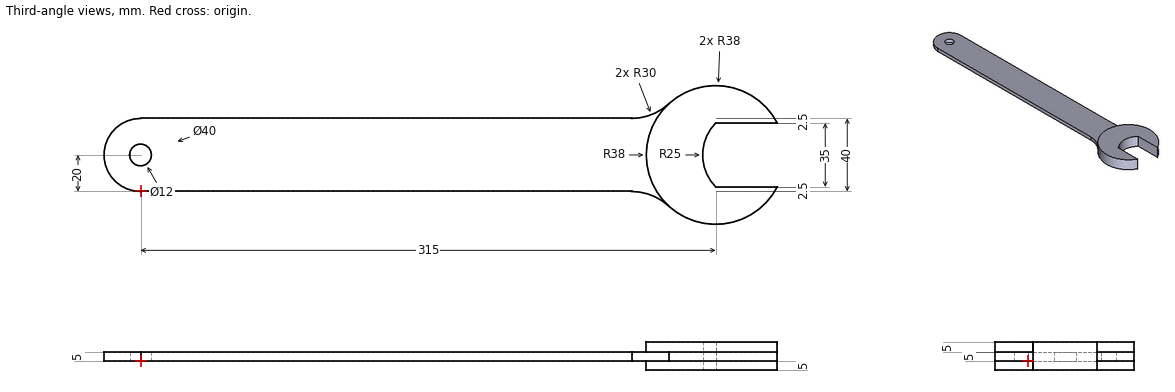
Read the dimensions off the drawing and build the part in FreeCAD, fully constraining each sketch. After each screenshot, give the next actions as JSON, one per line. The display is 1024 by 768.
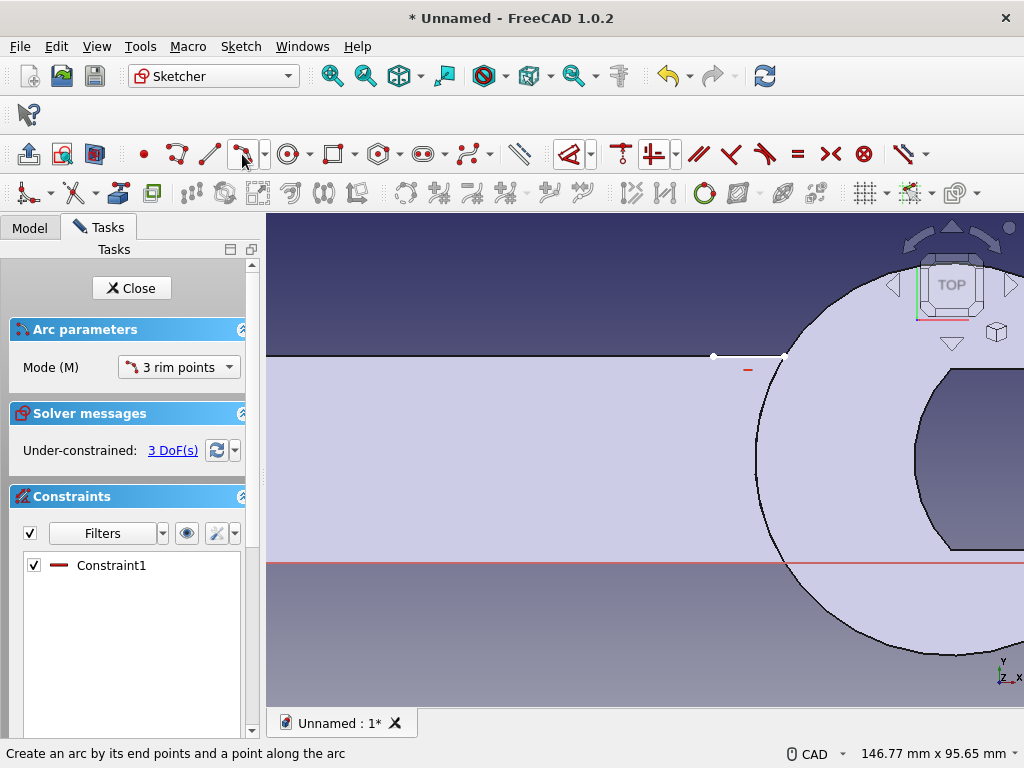
{"action": "left_click", "coordinate": [713, 357]}
{"action": "left_click", "coordinate": [818, 315]}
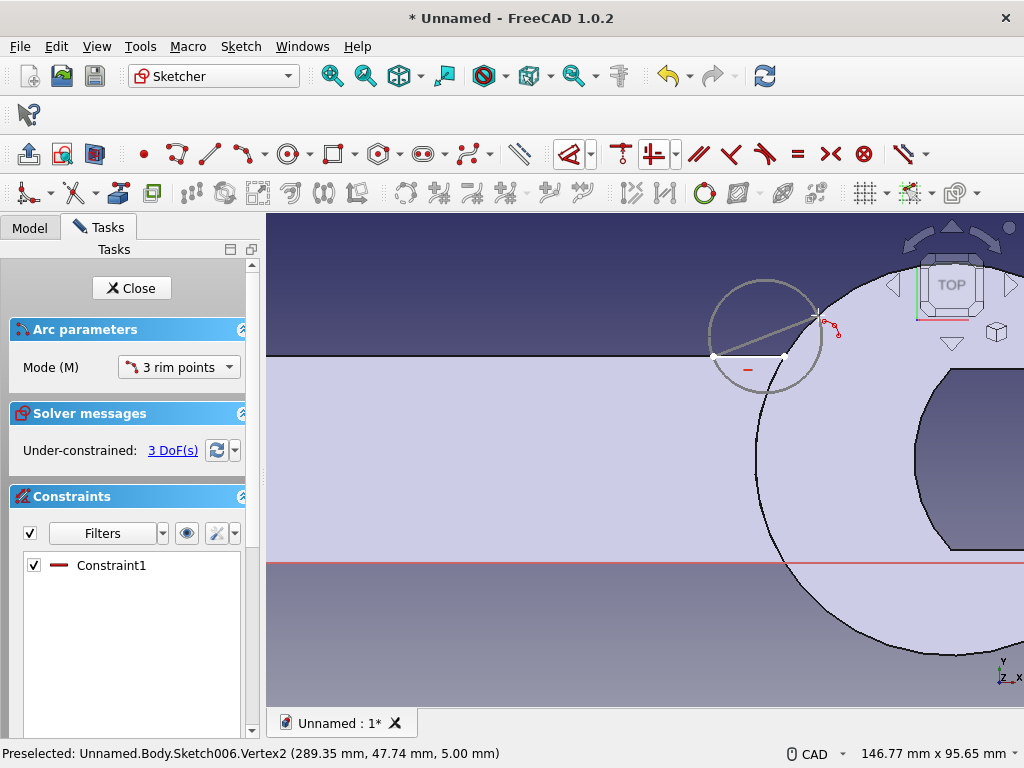
{"action": "scroll", "coordinate": [770, 345], "scroll_direction": "up", "scroll_amount": 3}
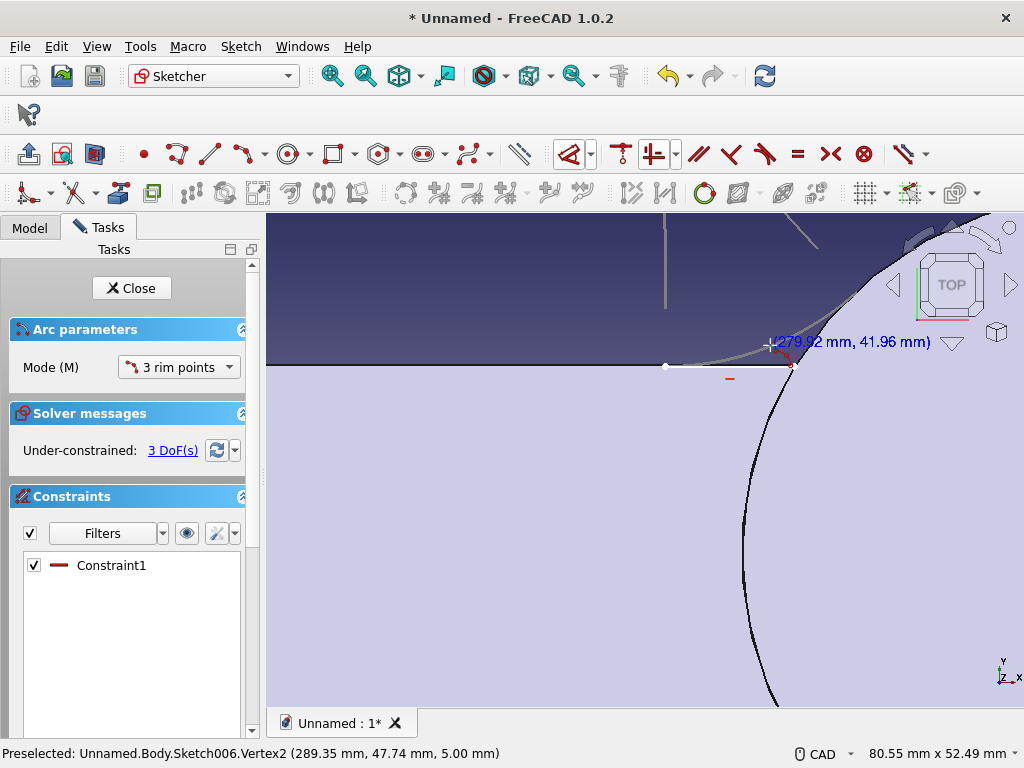
{"action": "left_click", "coordinate": [769, 346]}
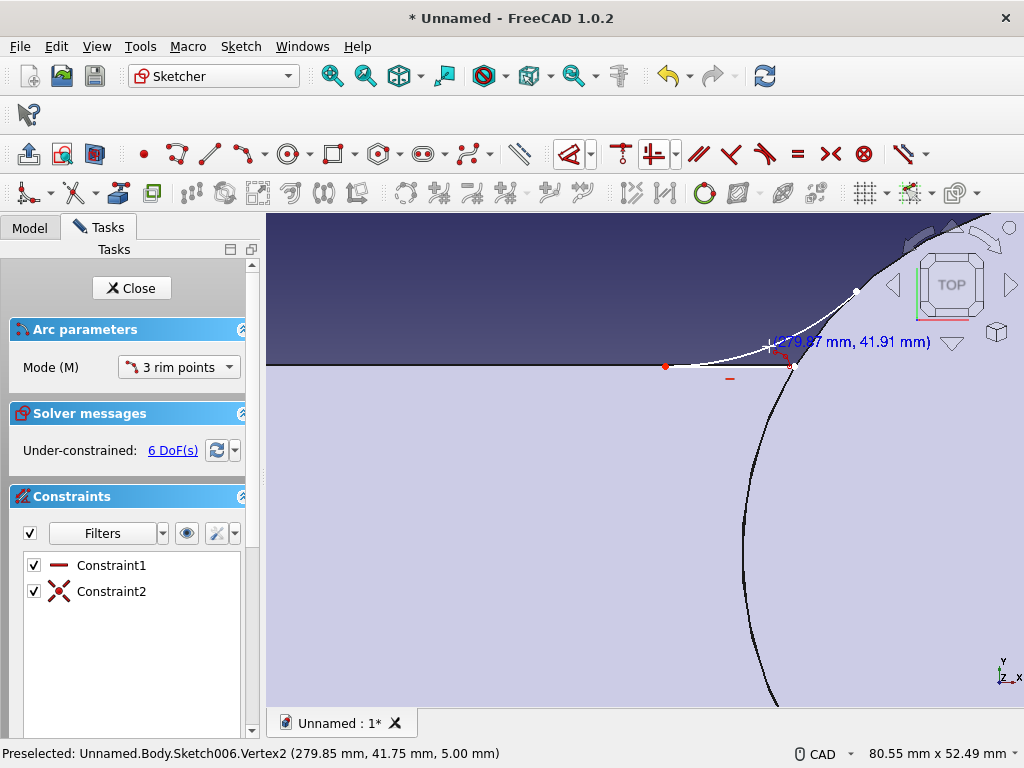
{"action": "left_click", "coordinate": [857, 292]}
{"action": "left_click", "coordinate": [795, 367]}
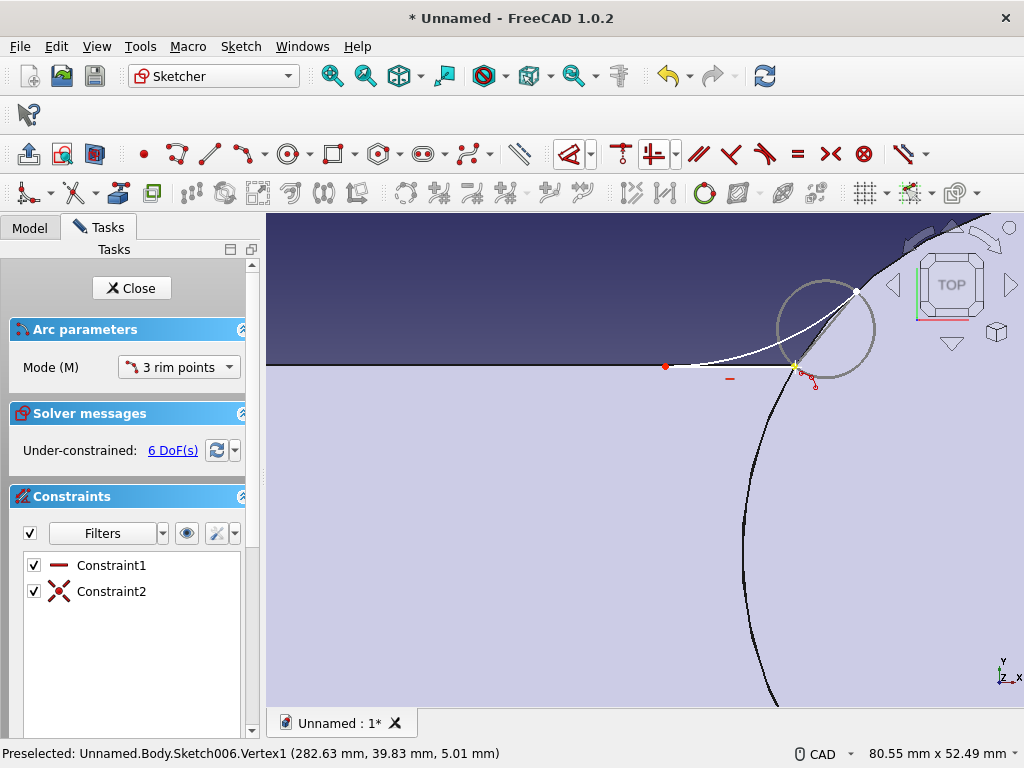
{"action": "scroll", "coordinate": [824, 326], "scroll_direction": "up", "scroll_amount": 8}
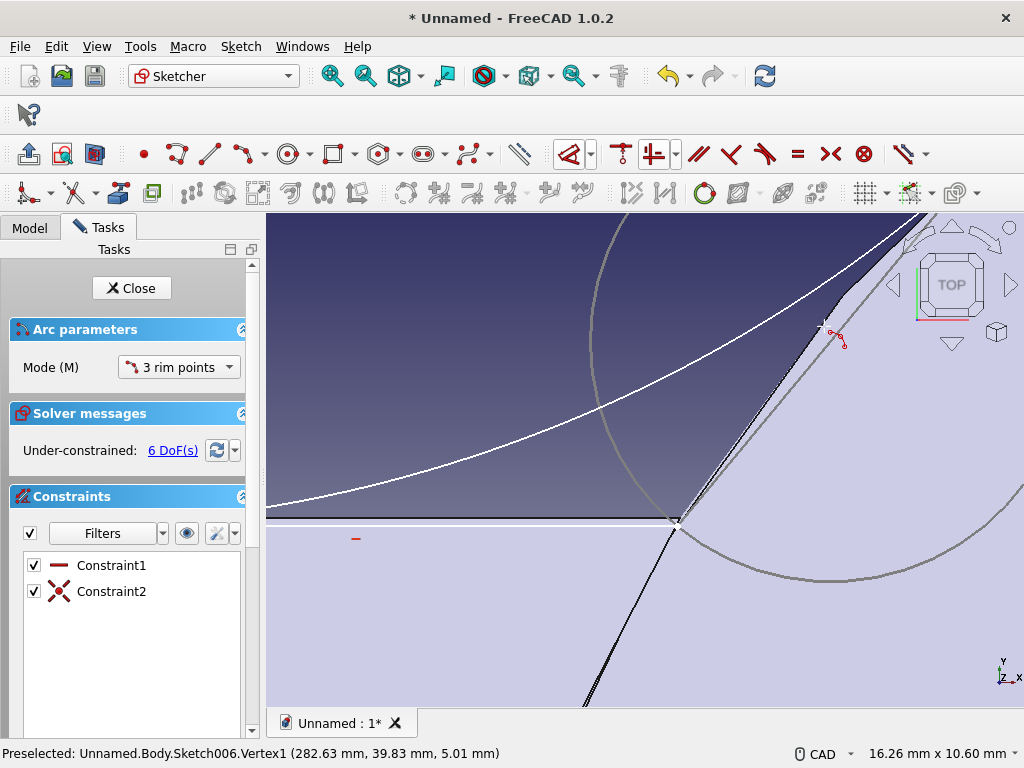
{"action": "left_click", "coordinate": [820, 323]}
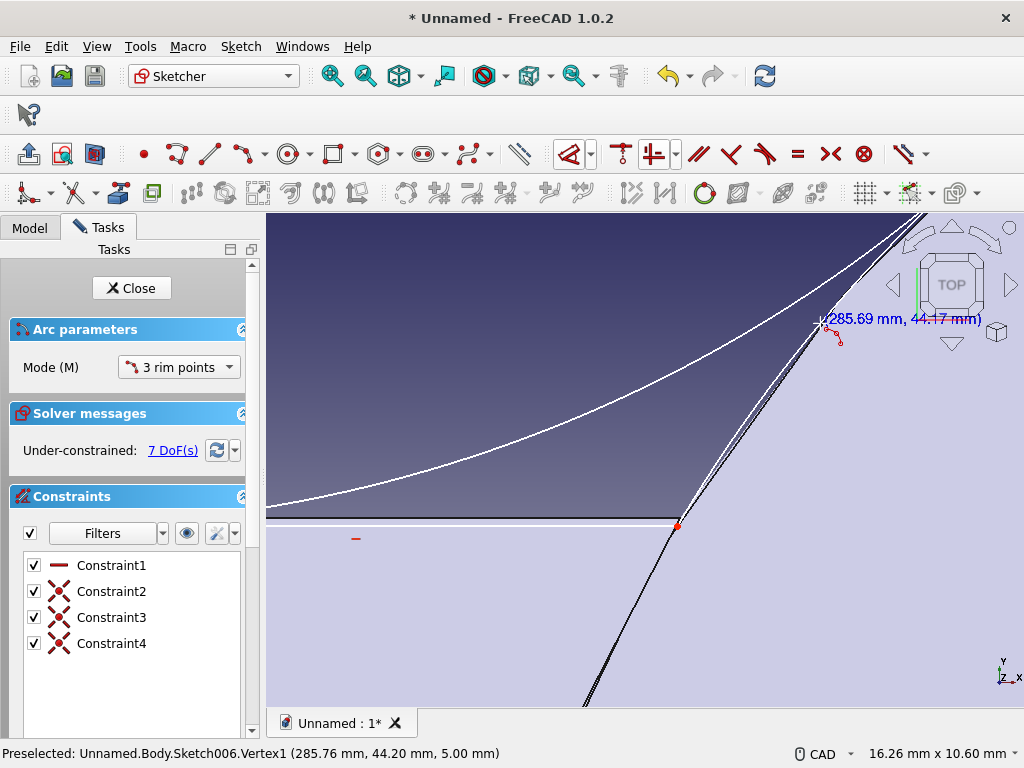
{"action": "left_click", "coordinate": [210, 154]}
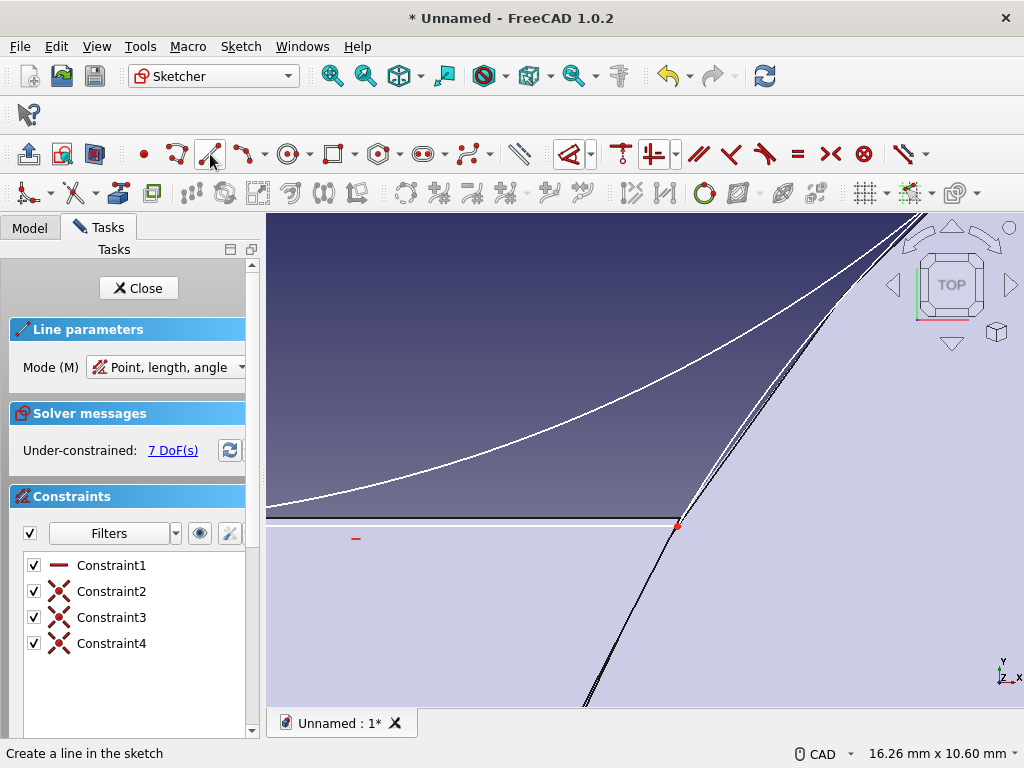
{"action": "scroll", "coordinate": [585, 337], "scroll_direction": "down", "scroll_amount": 11}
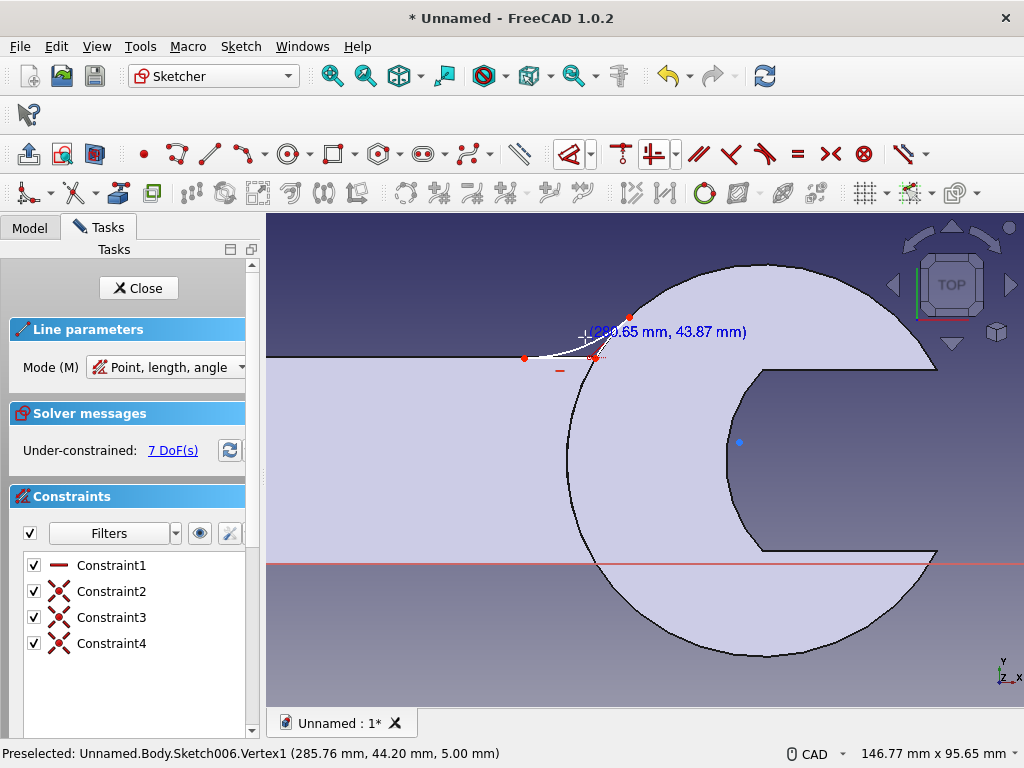
{"action": "left_click", "coordinate": [525, 564]}
{"action": "left_click", "coordinate": [596, 555]}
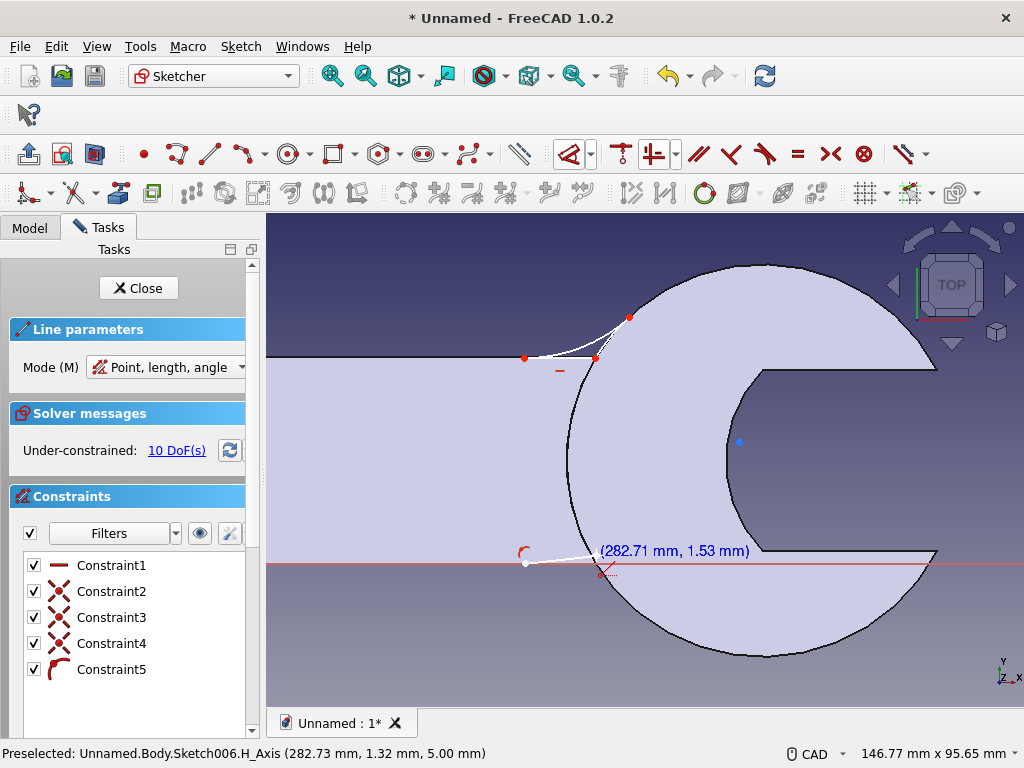
{"action": "left_click", "coordinate": [242, 154]}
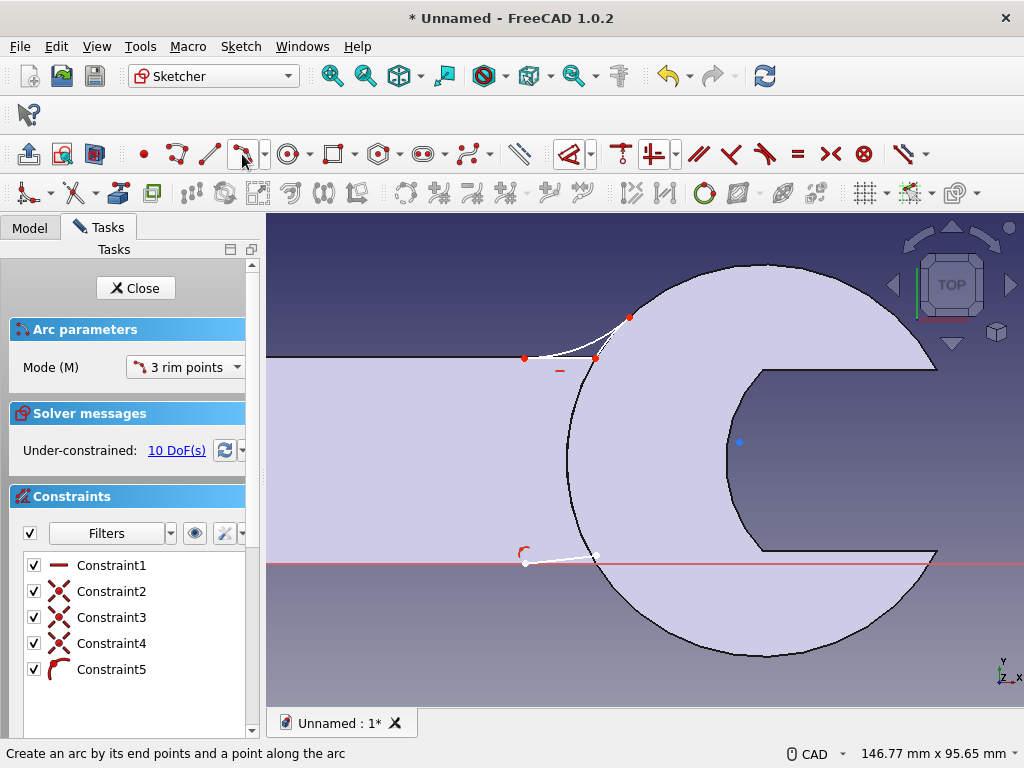
{"action": "left_click", "coordinate": [596, 556]}
{"action": "left_click", "coordinate": [630, 605]}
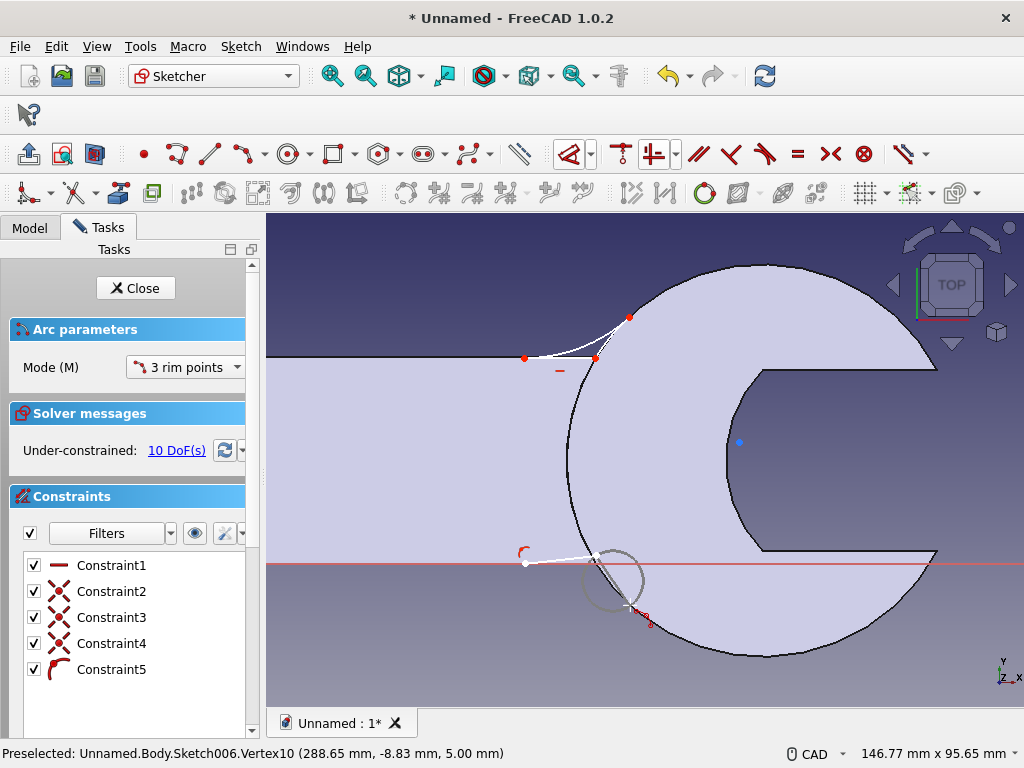
{"action": "scroll", "coordinate": [611, 586], "scroll_direction": "up", "scroll_amount": 11}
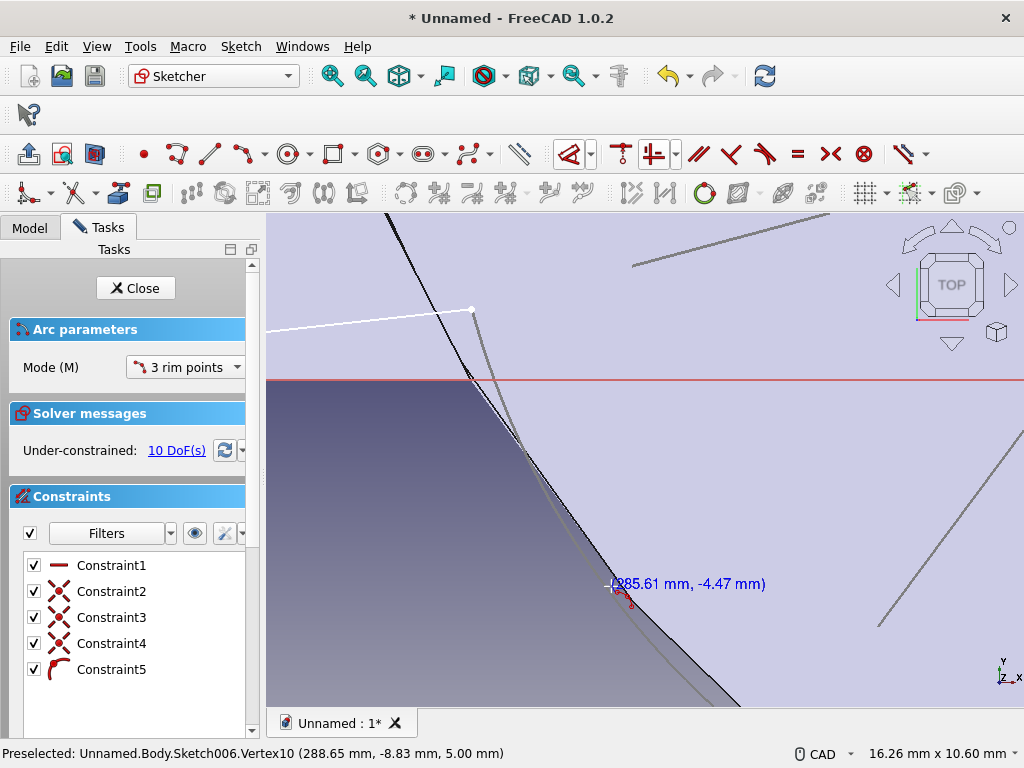
{"action": "left_click", "coordinate": [611, 576]}